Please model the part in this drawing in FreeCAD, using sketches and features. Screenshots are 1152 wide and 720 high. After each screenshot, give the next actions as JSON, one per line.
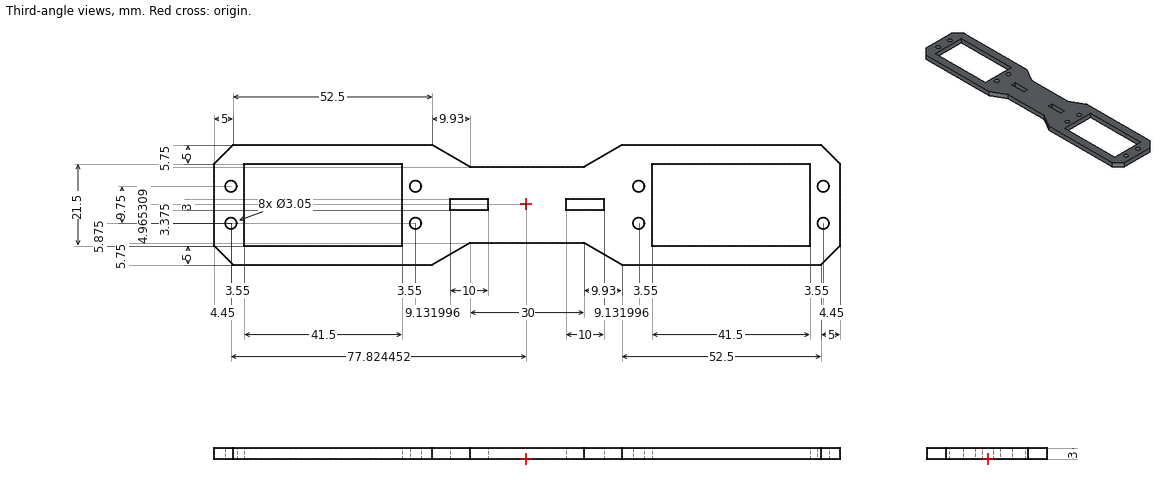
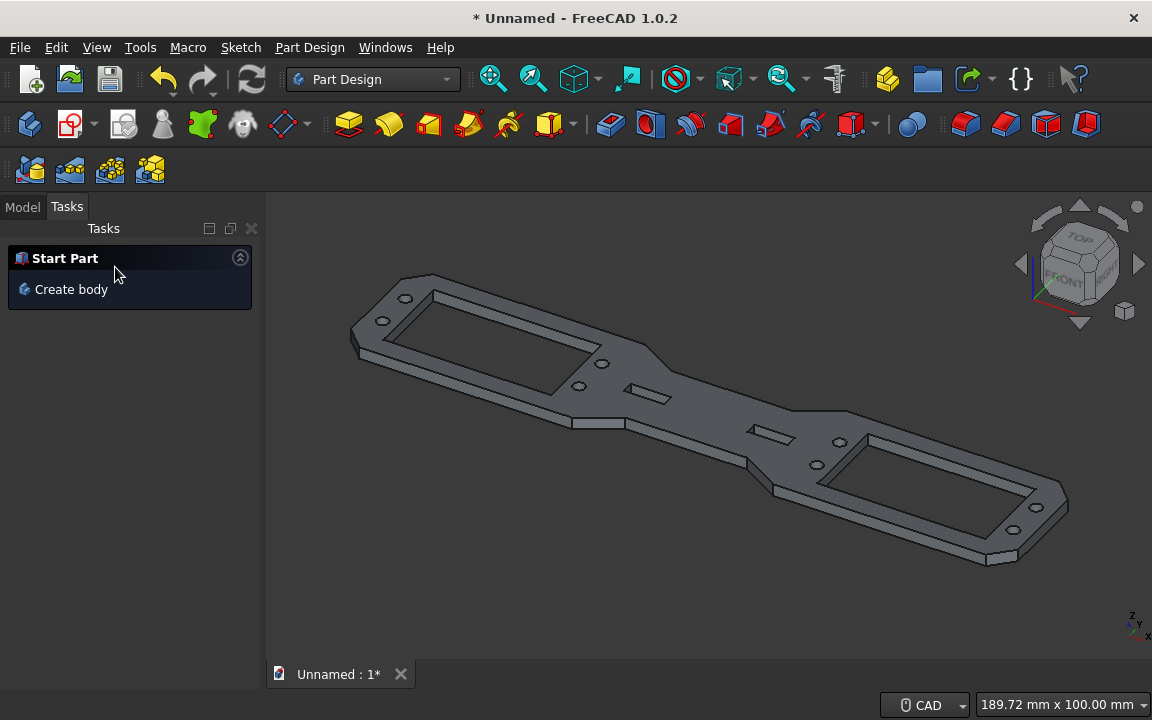
{"action": "key", "text": "0"}